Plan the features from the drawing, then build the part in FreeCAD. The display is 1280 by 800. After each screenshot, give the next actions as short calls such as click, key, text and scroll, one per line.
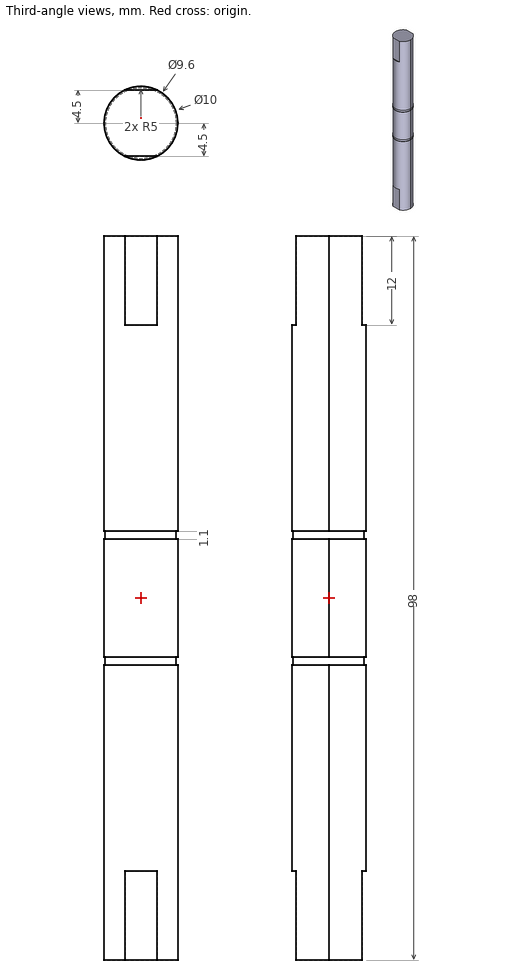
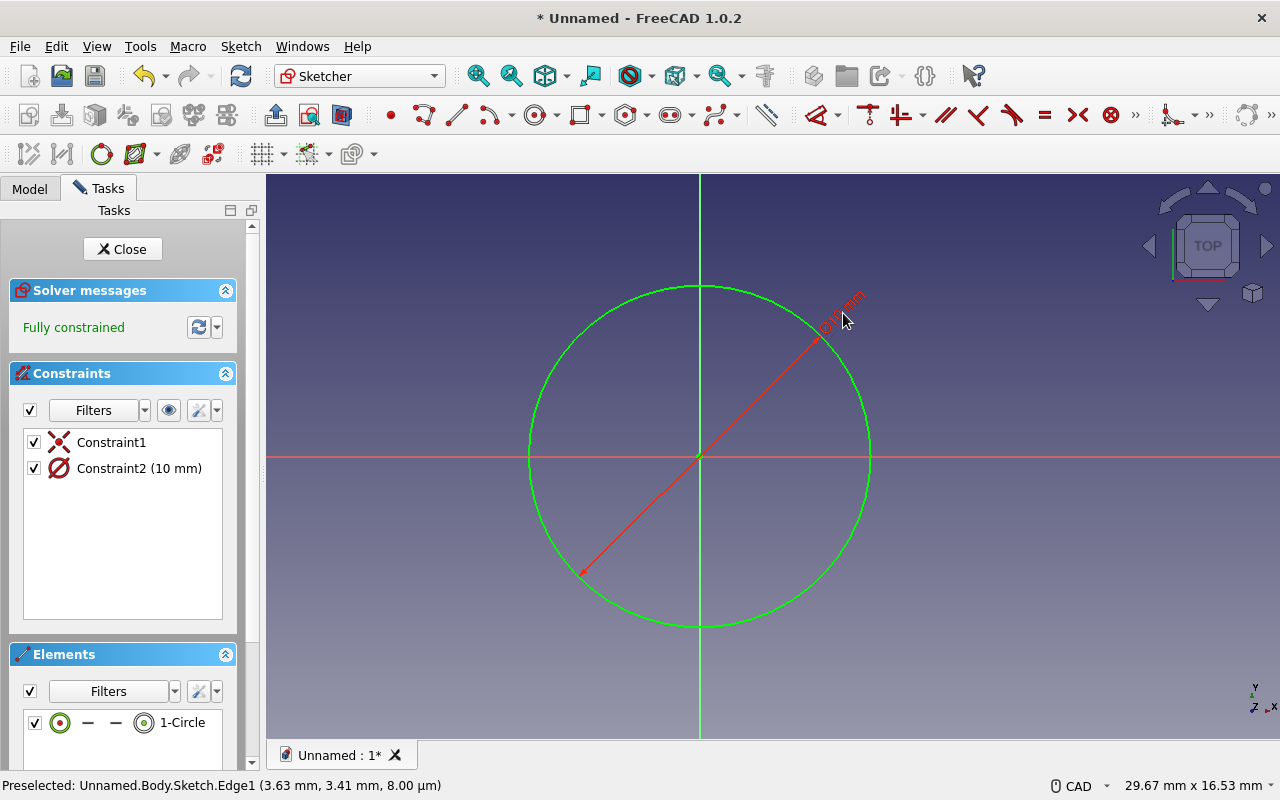
click(123, 249)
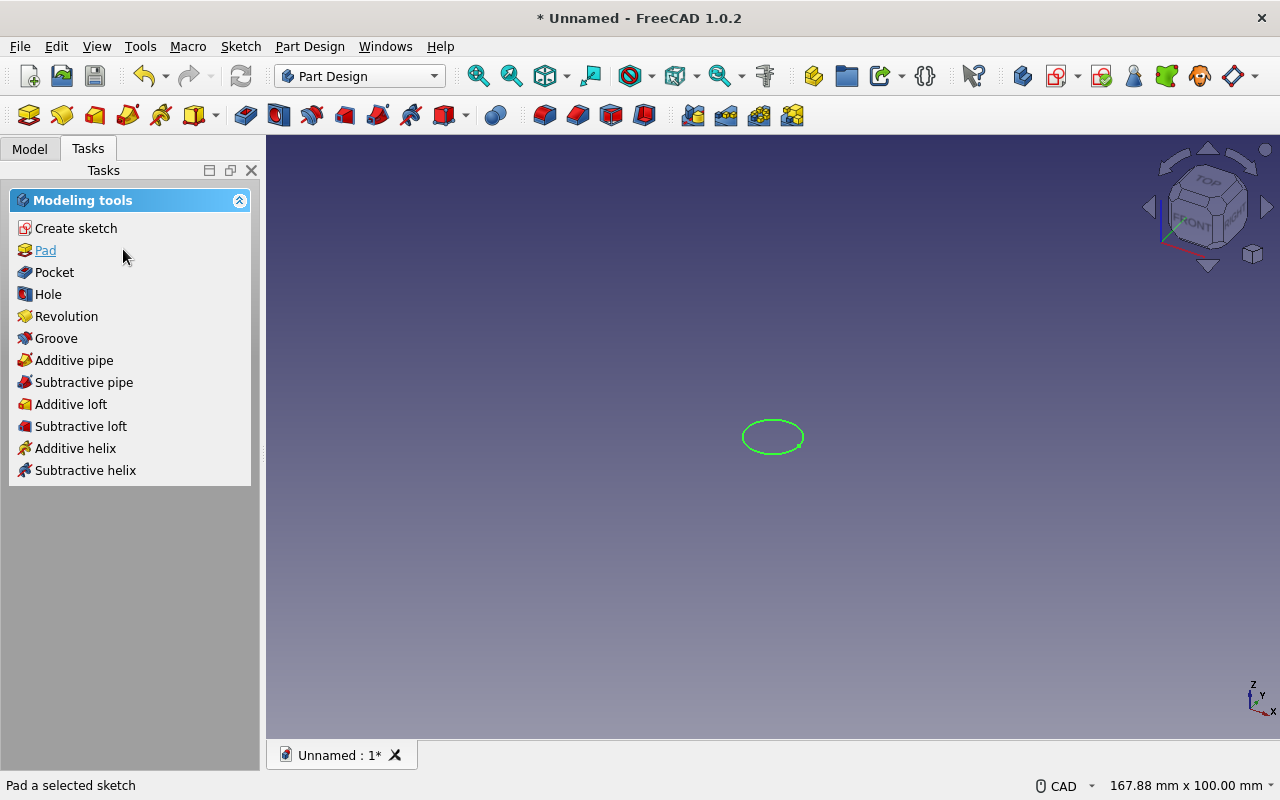
click(29, 116)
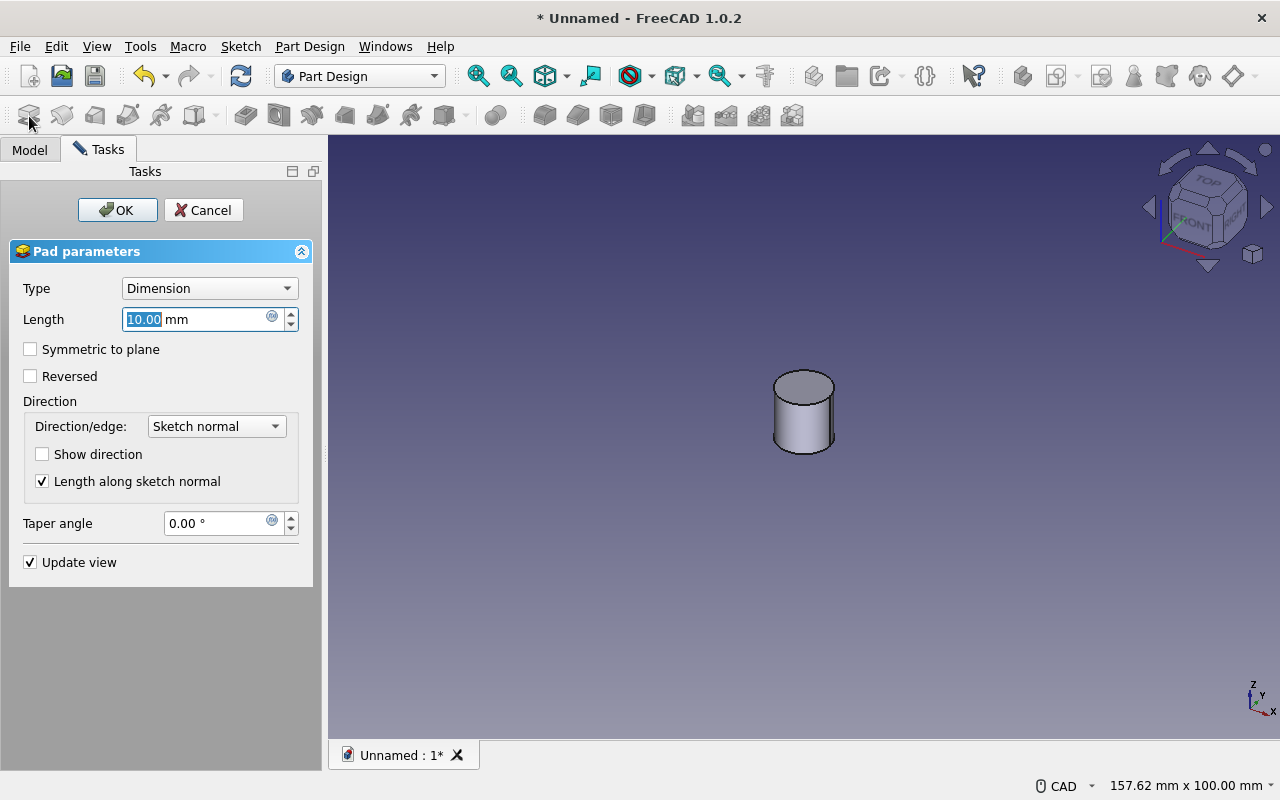
text(98)
key(Tab)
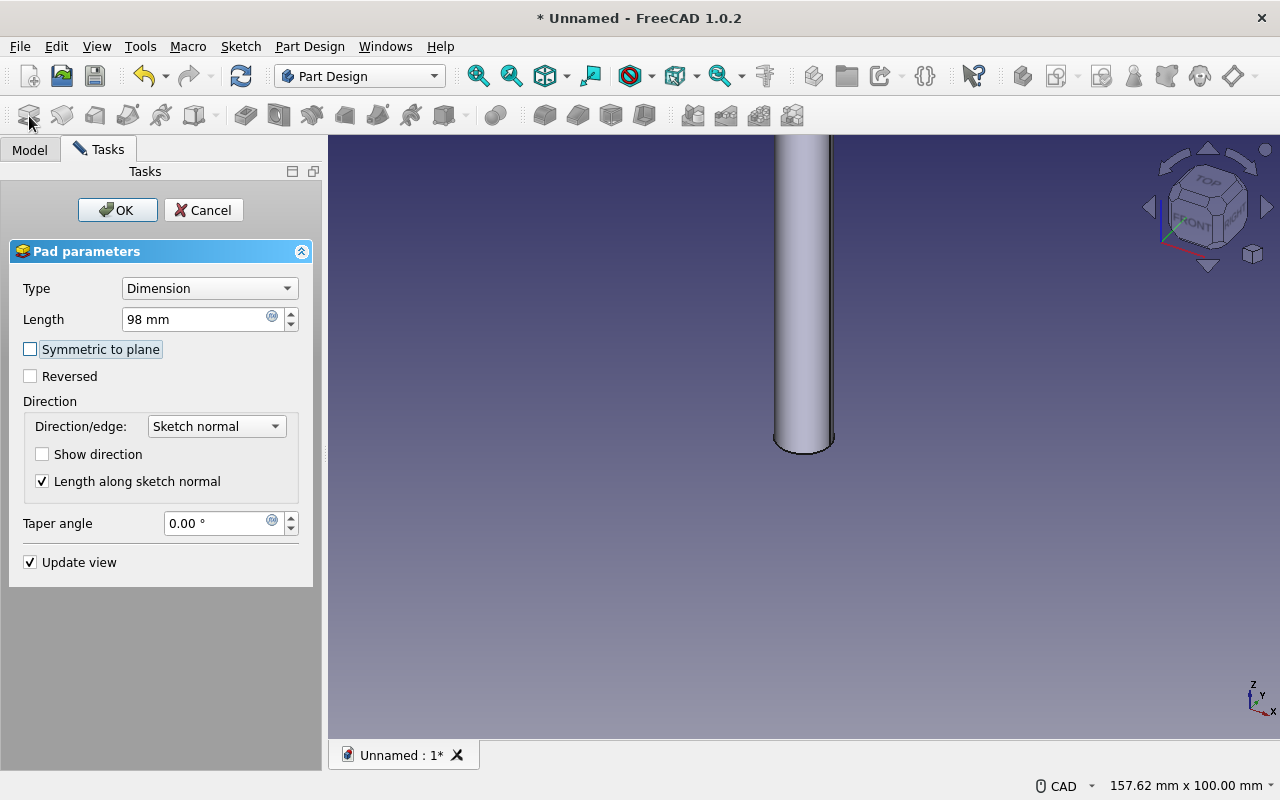
click(31, 349)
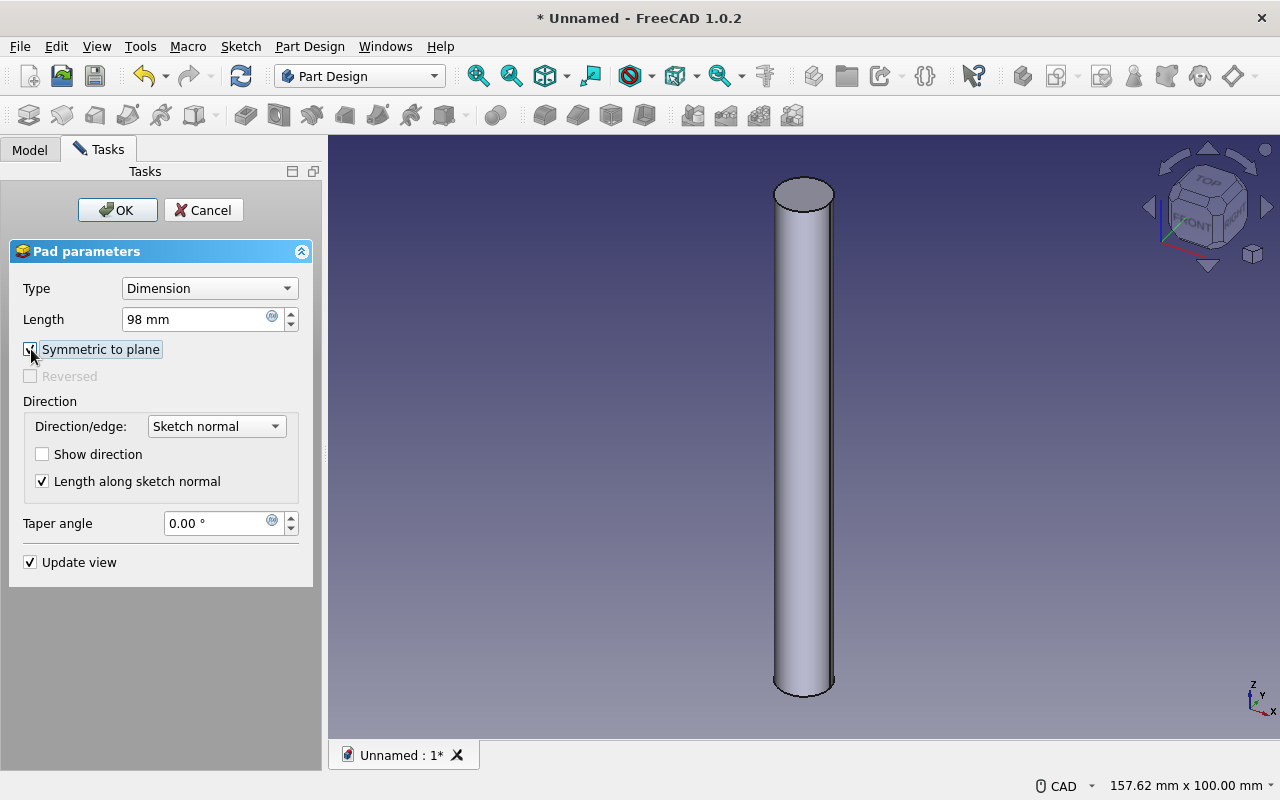
click(118, 210)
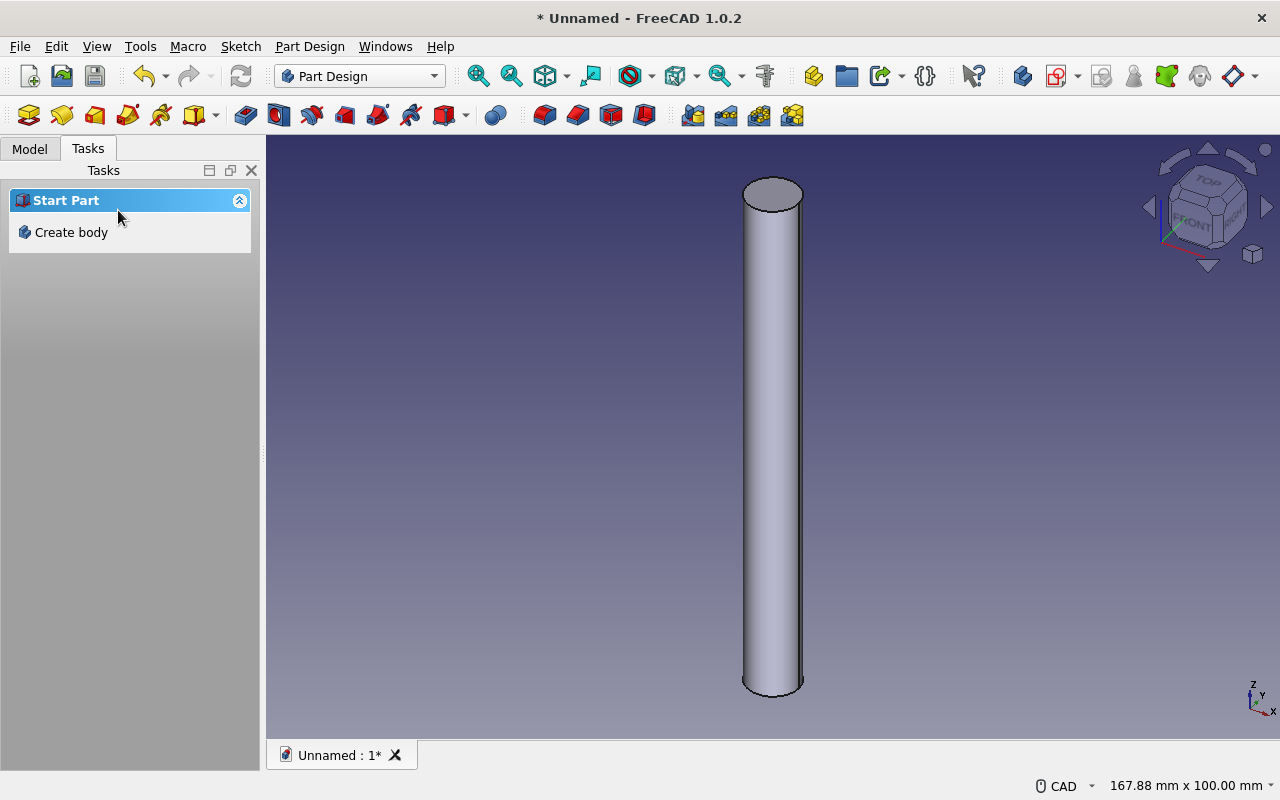
click(30, 148)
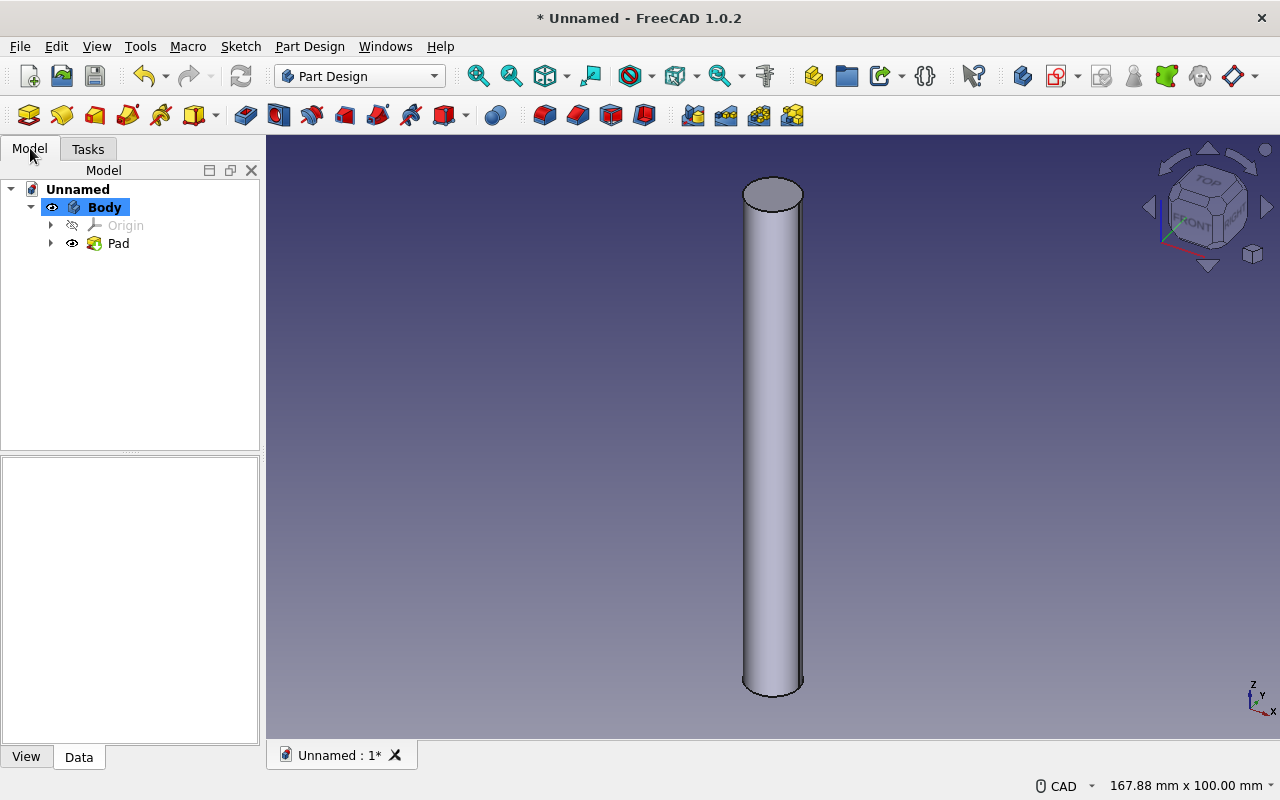
click(51, 225)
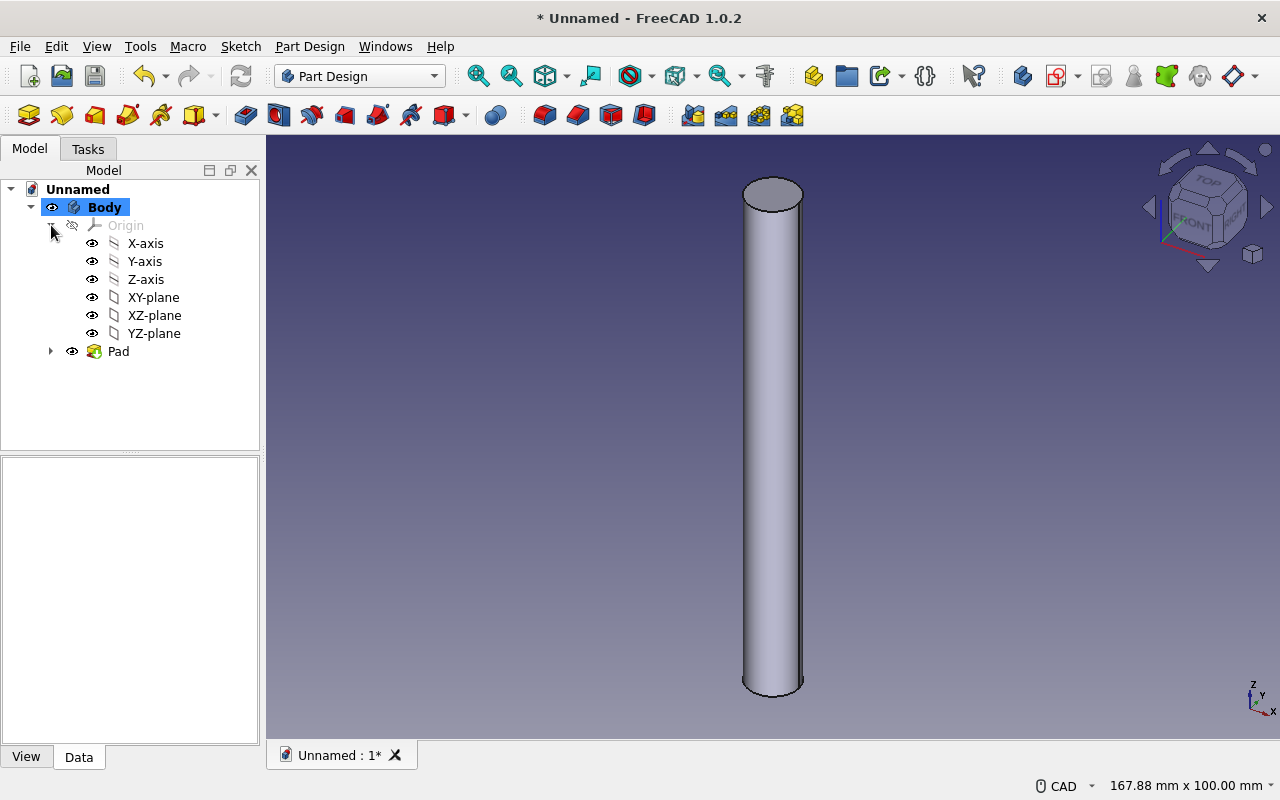
click(137, 297)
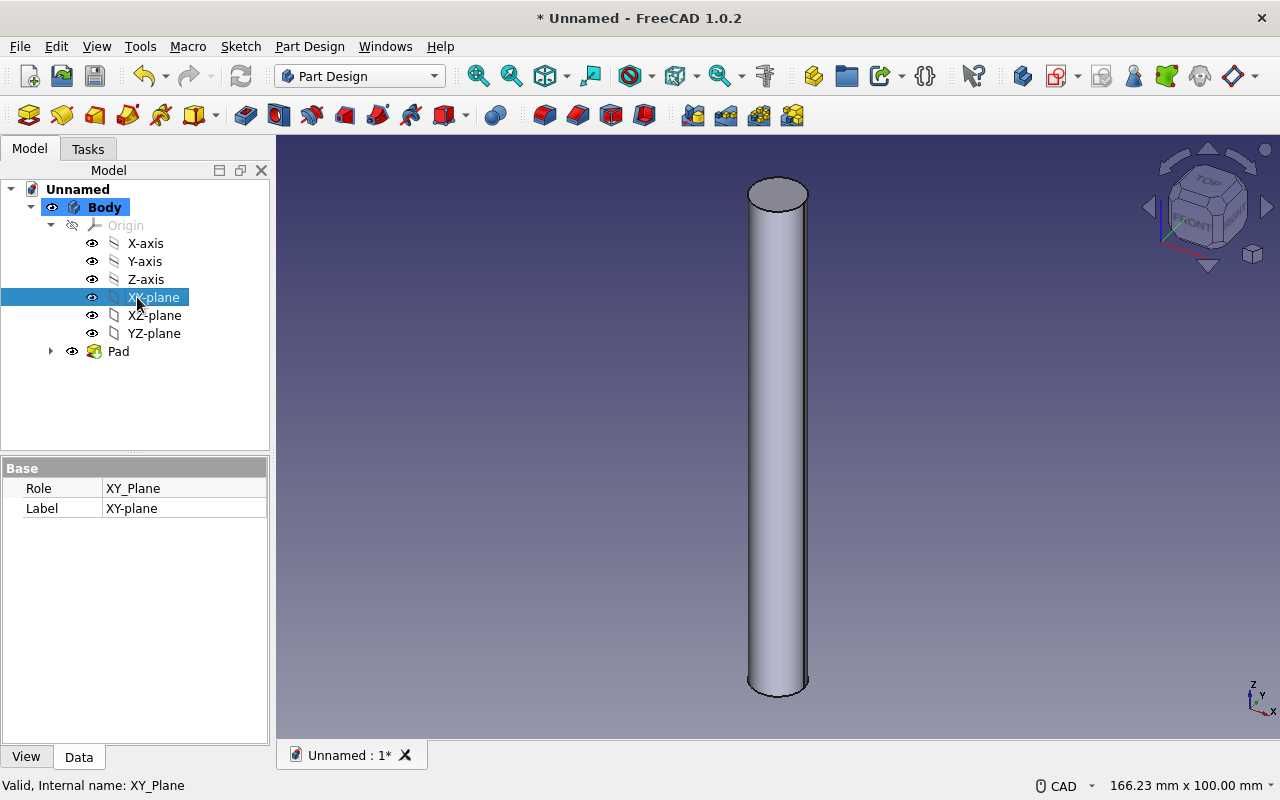
click(1232, 76)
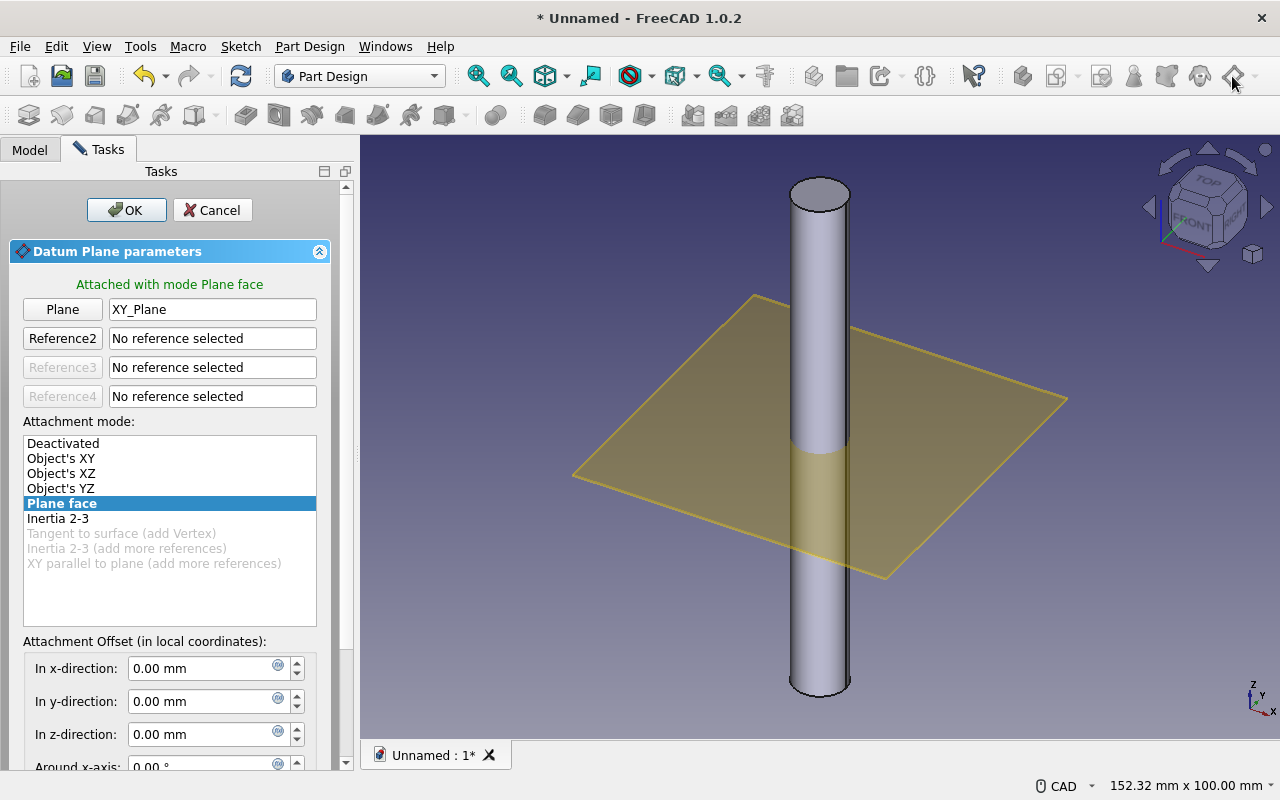
triple_click(210, 734)